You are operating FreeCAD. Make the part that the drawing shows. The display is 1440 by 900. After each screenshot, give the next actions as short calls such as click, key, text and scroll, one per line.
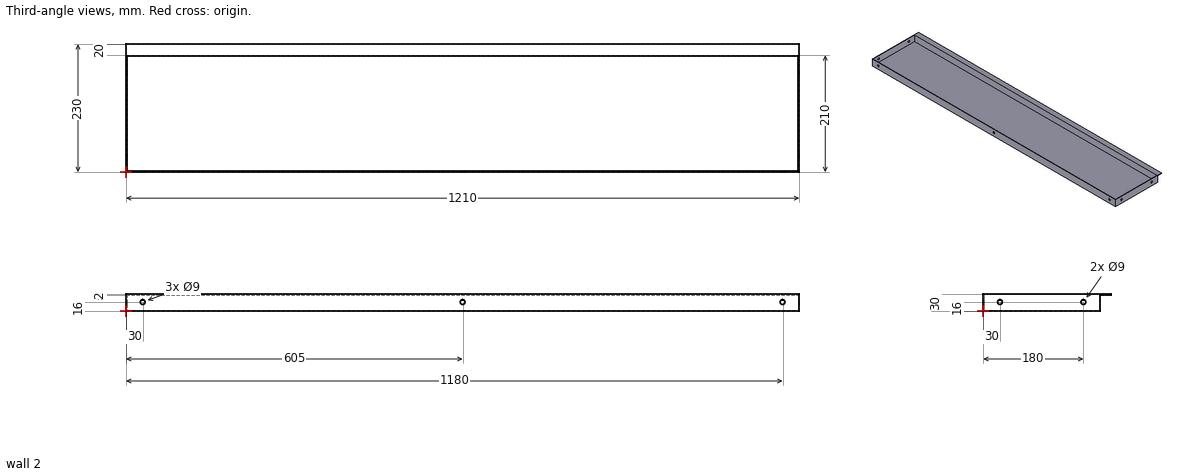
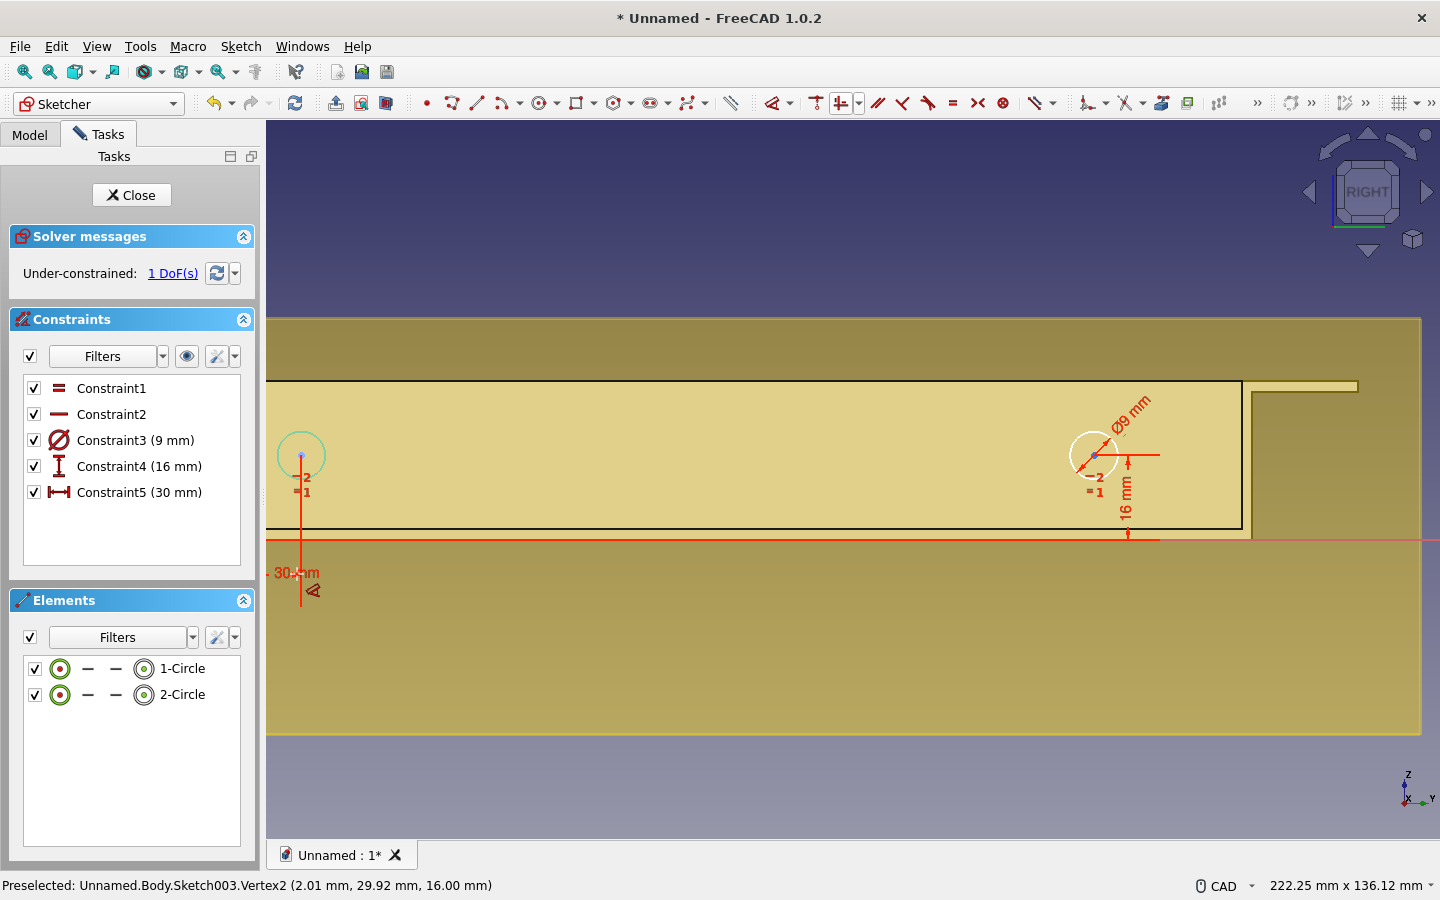
click(1094, 455)
click(694, 574)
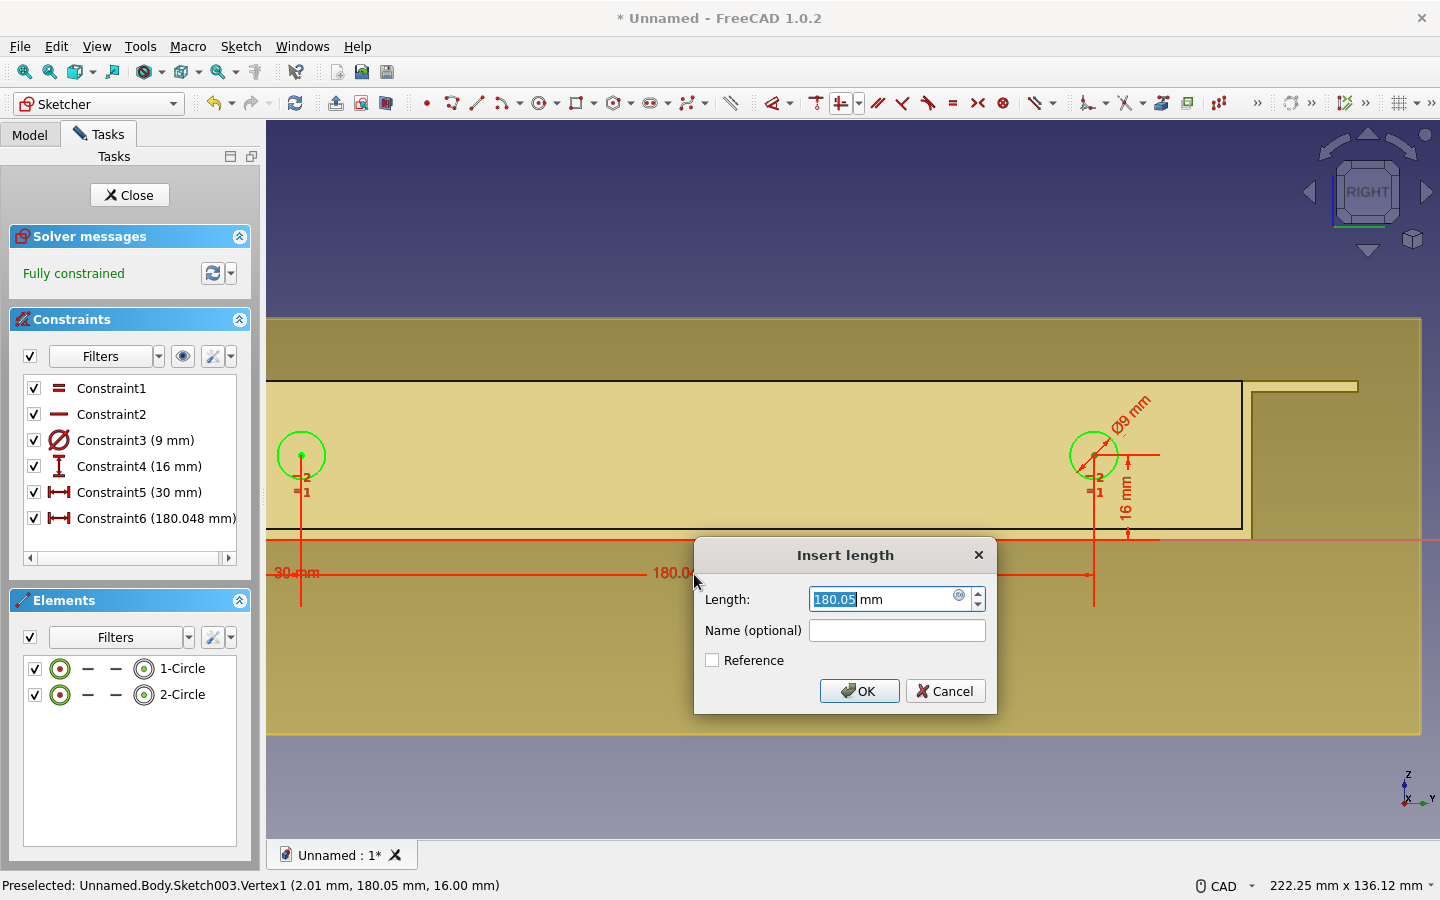
text(180)
key(Return)
key(Escape)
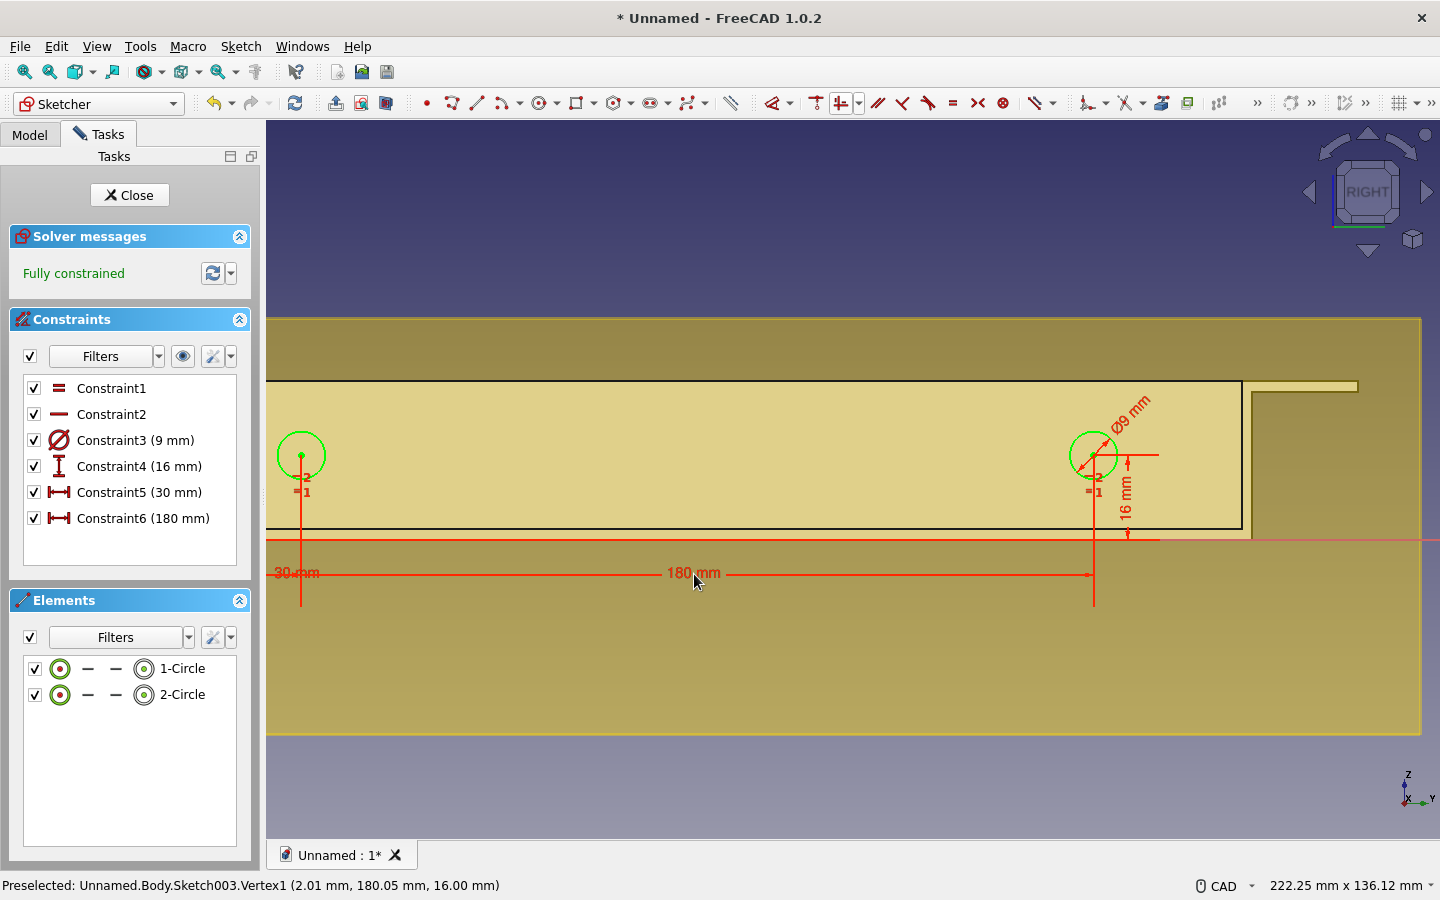
click(130, 195)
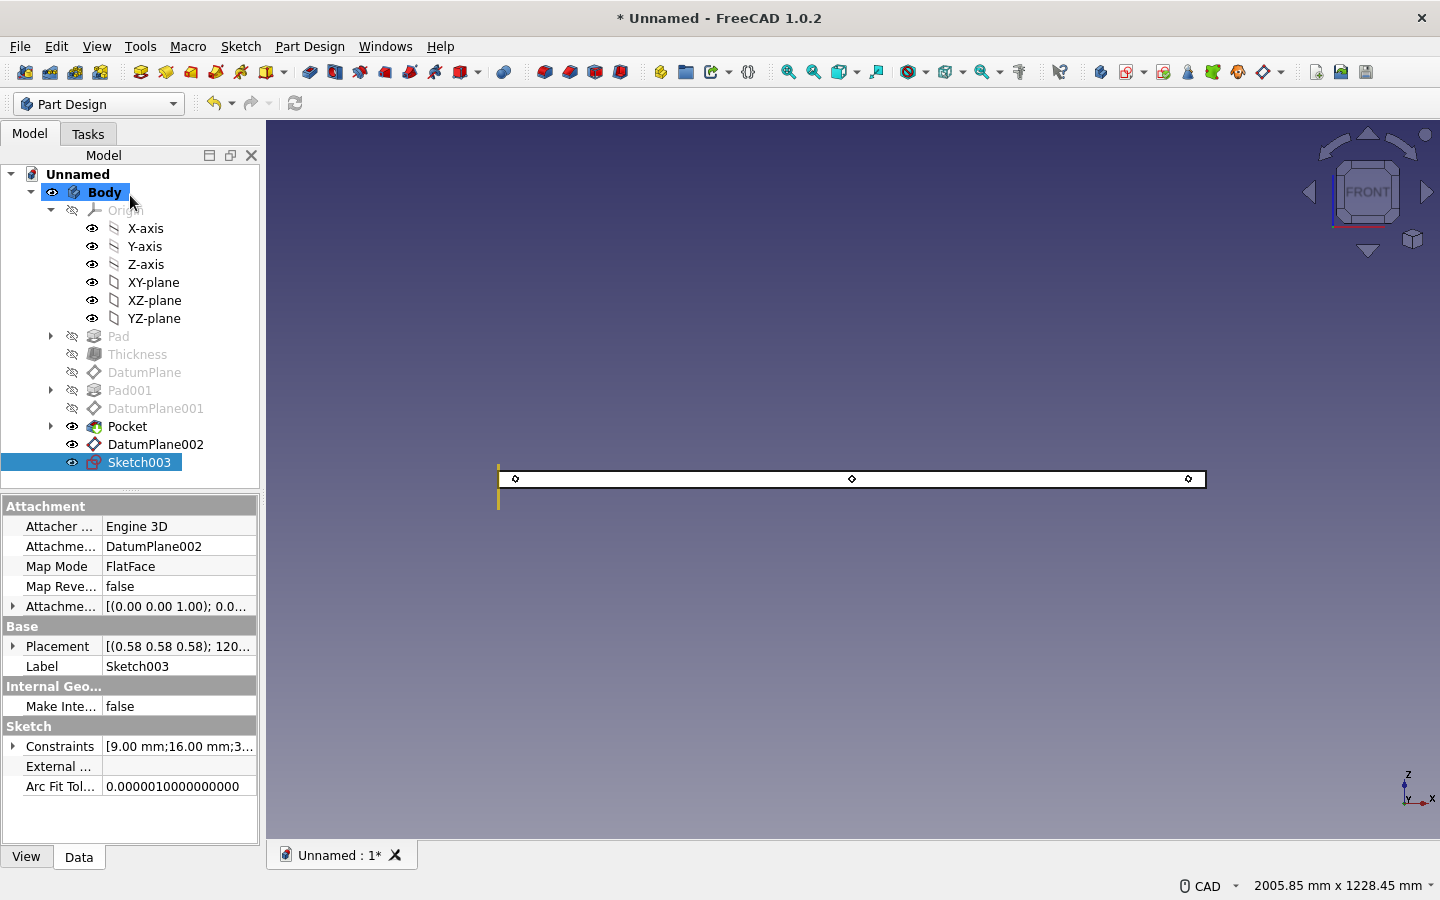
click(310, 72)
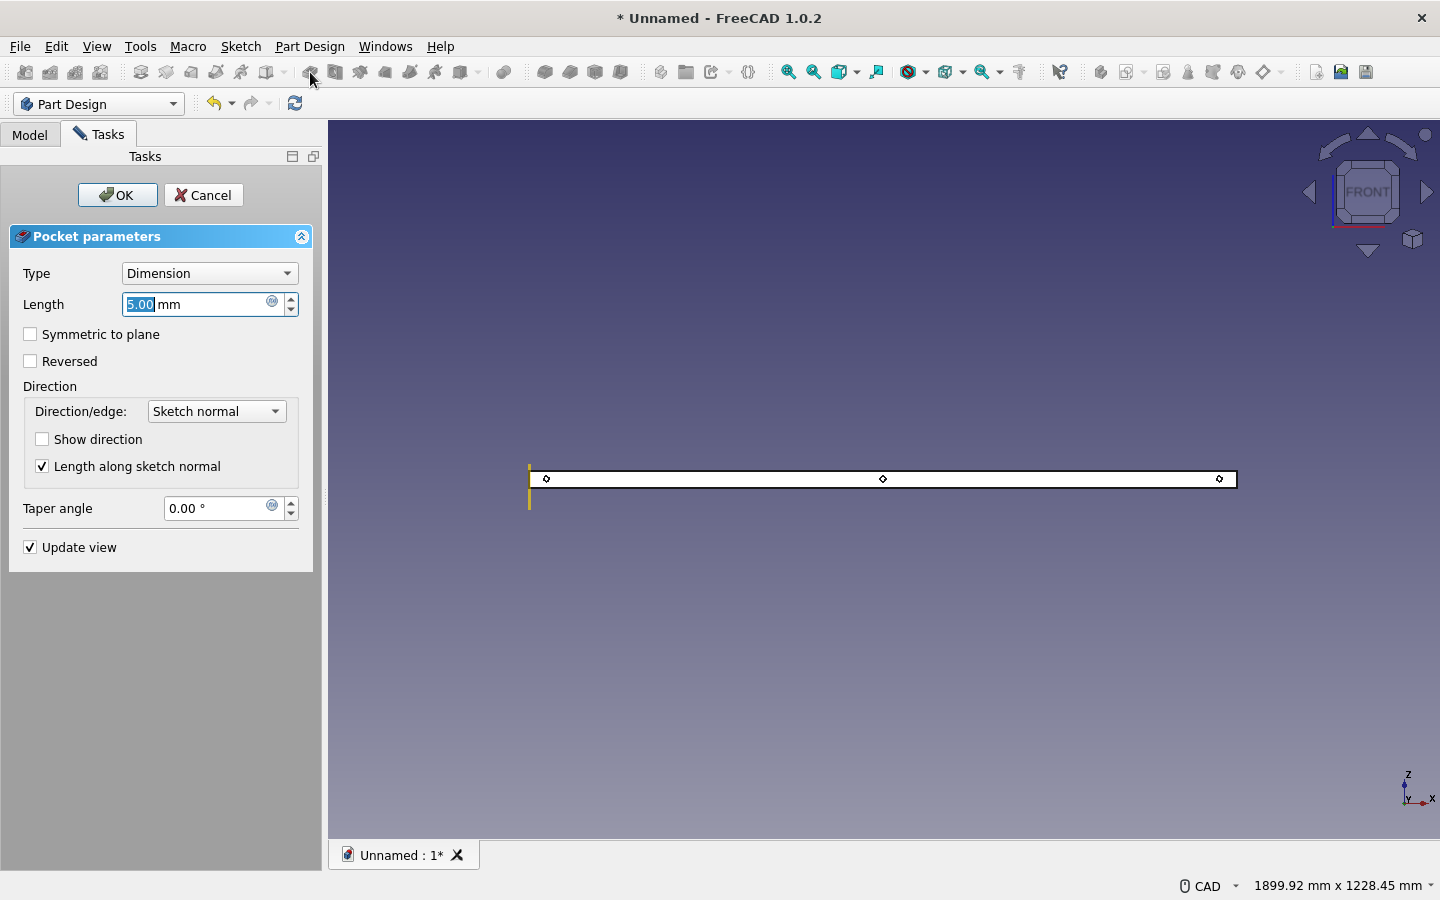
click(210, 274)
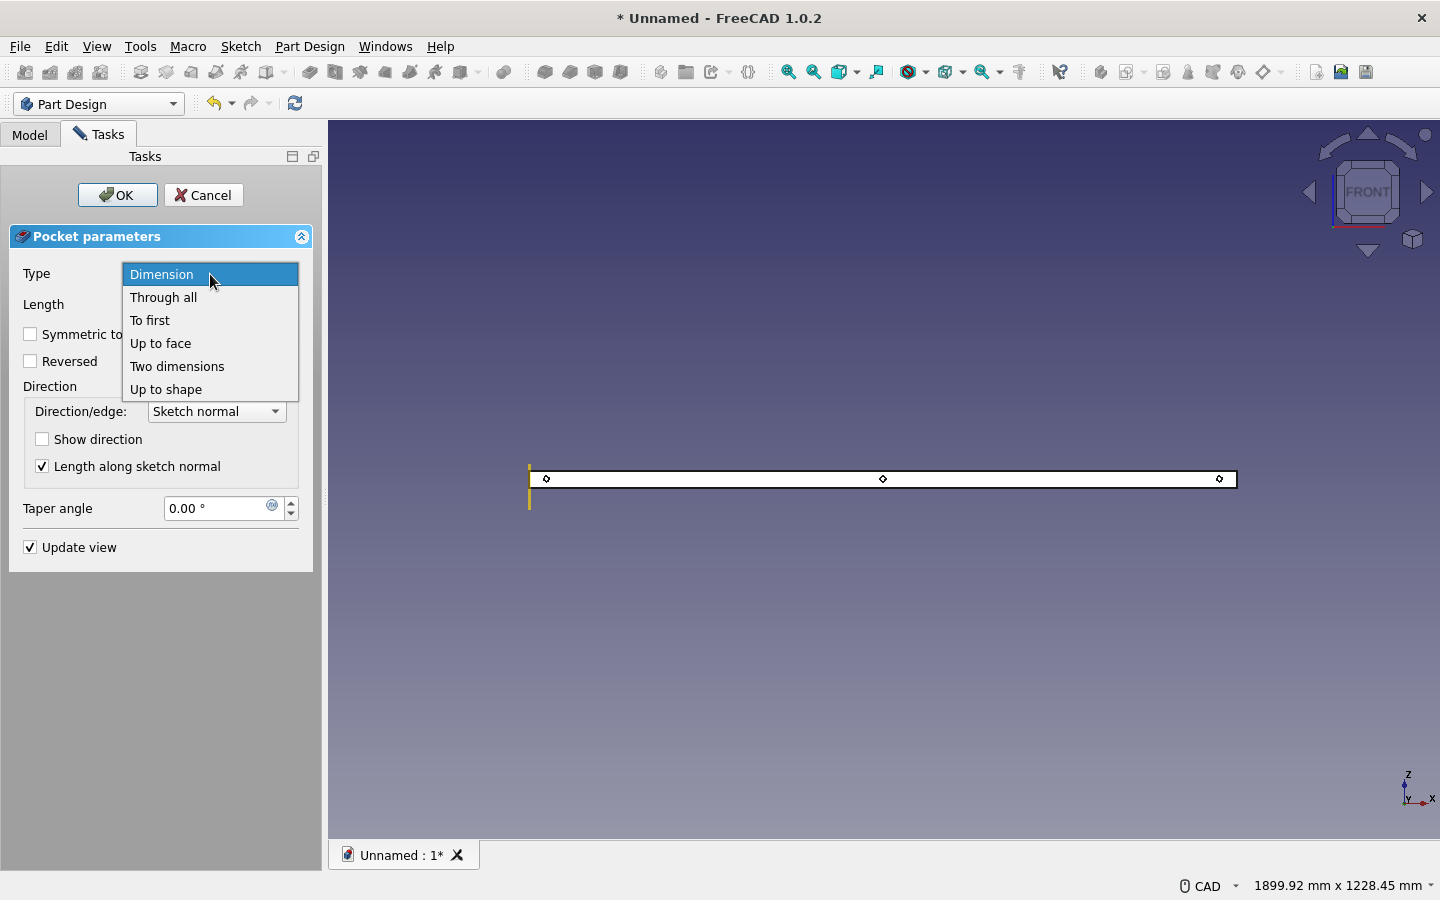
click(208, 366)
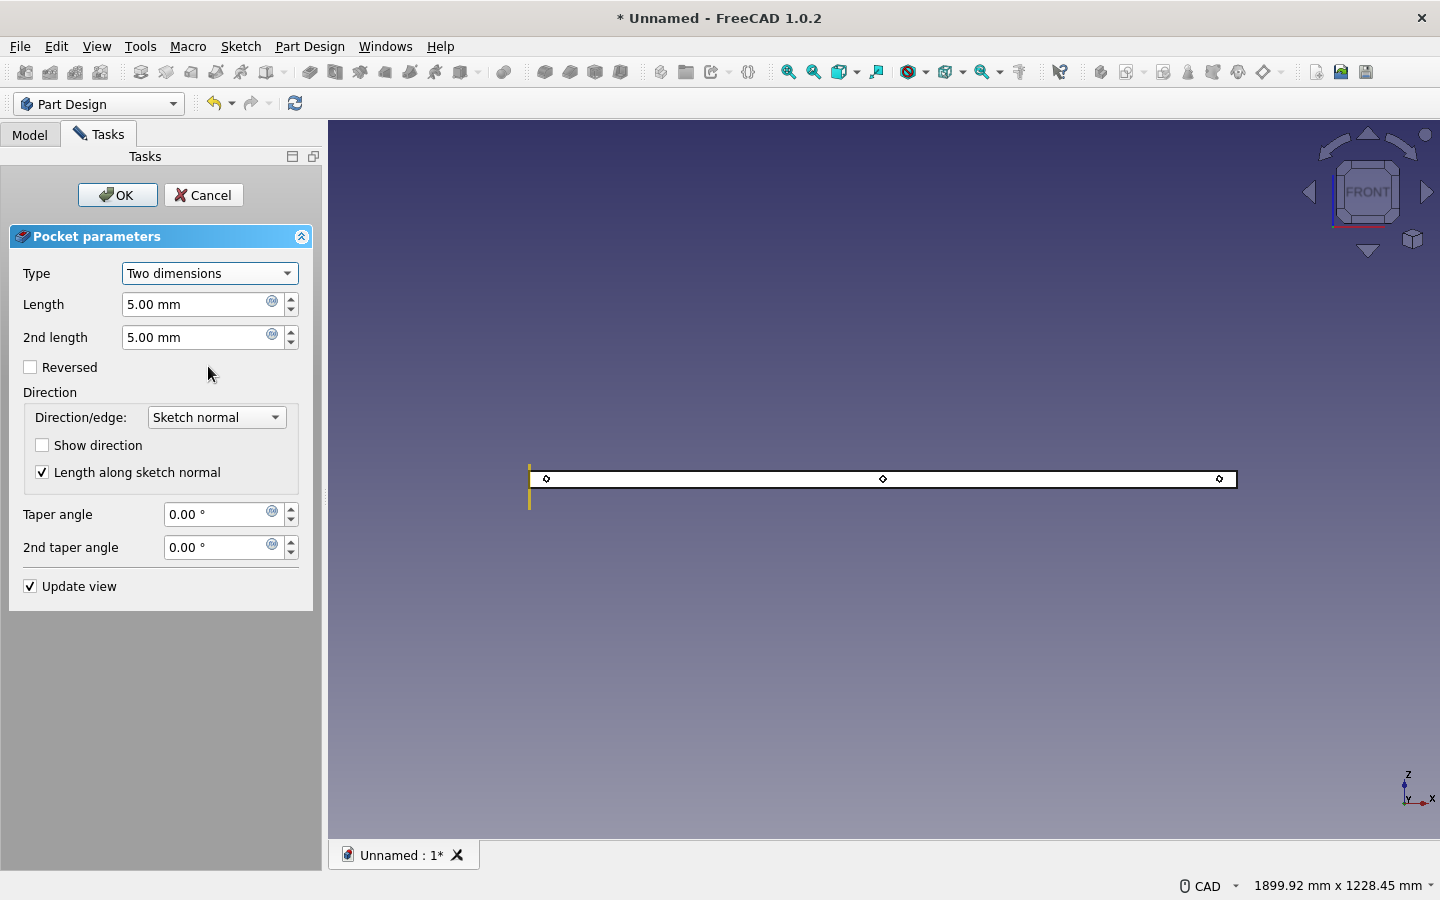
triple_click(204, 304)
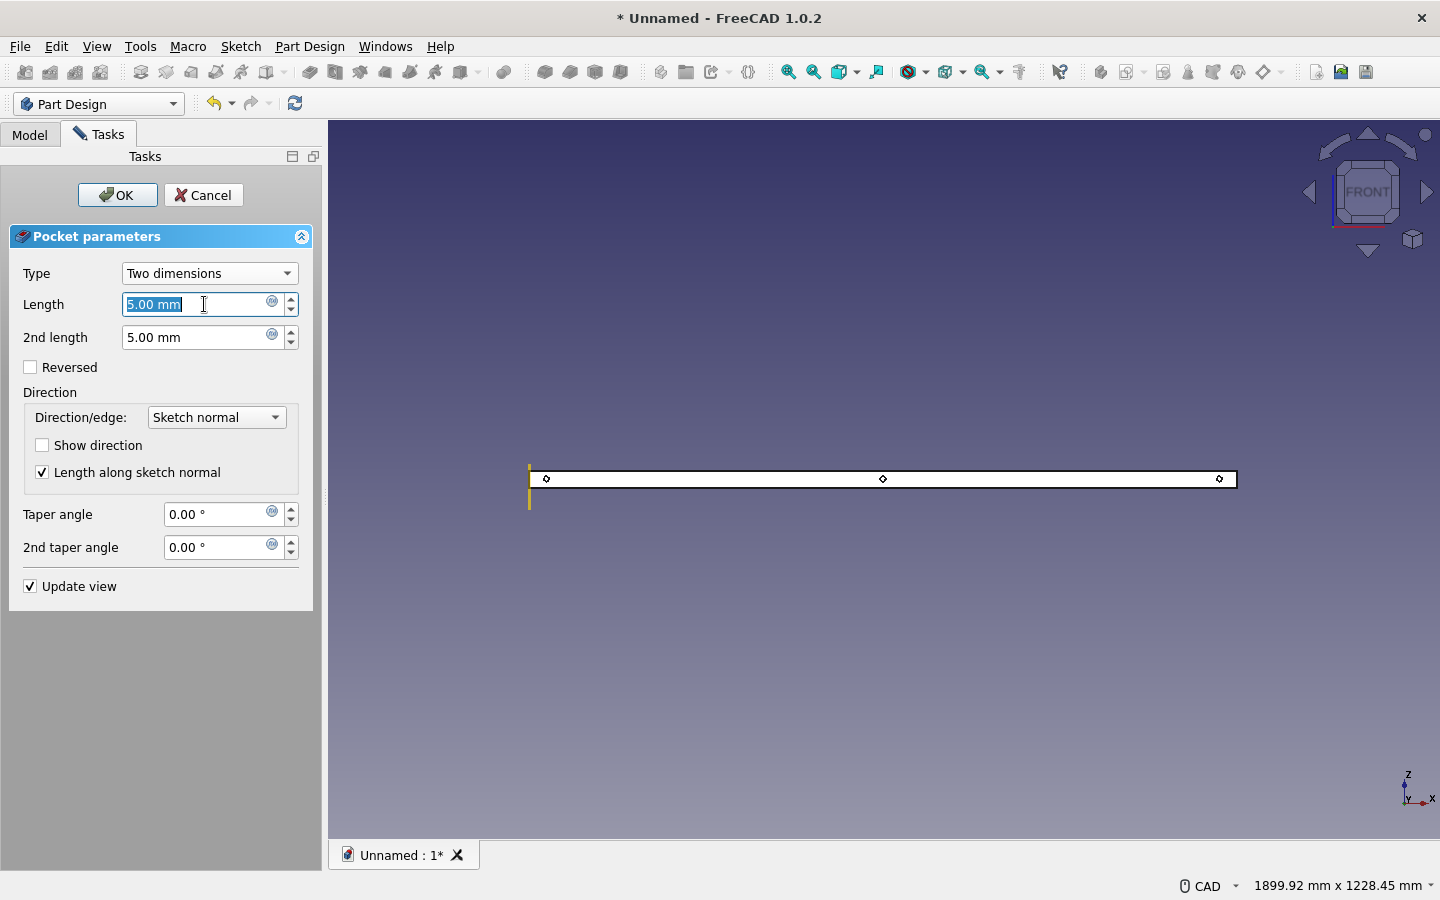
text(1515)
key(Tab)